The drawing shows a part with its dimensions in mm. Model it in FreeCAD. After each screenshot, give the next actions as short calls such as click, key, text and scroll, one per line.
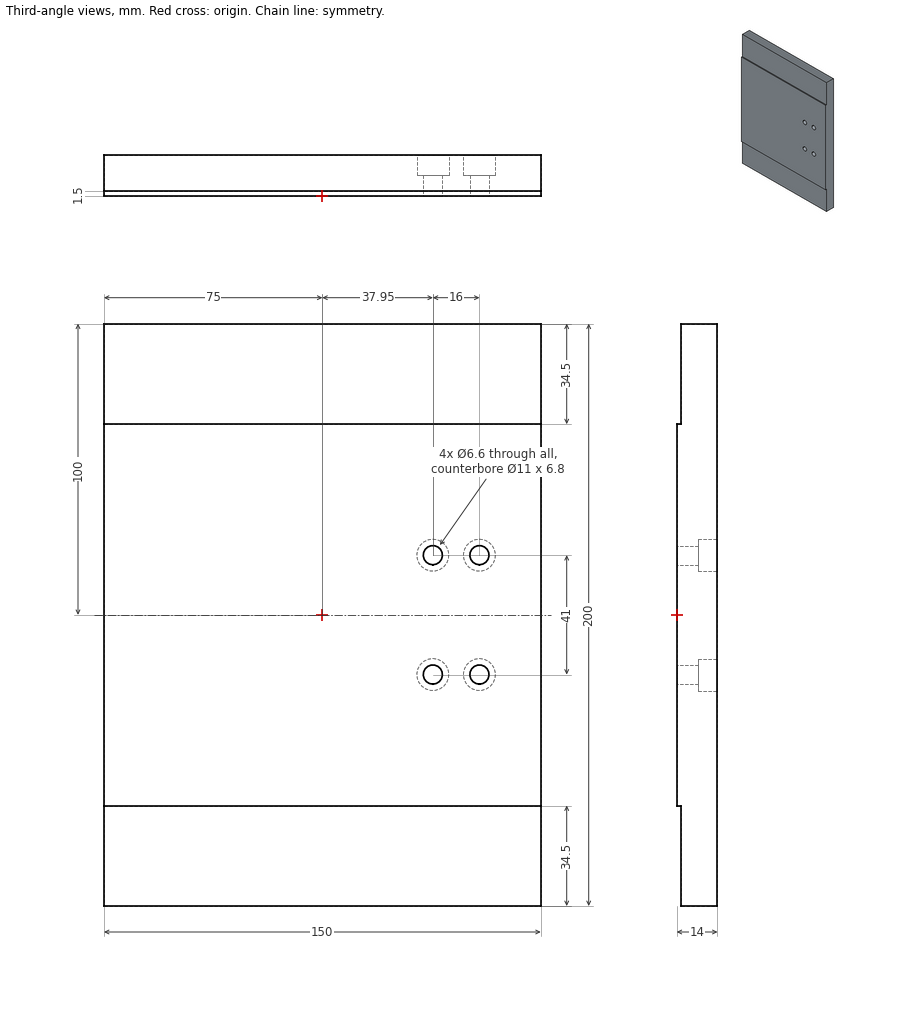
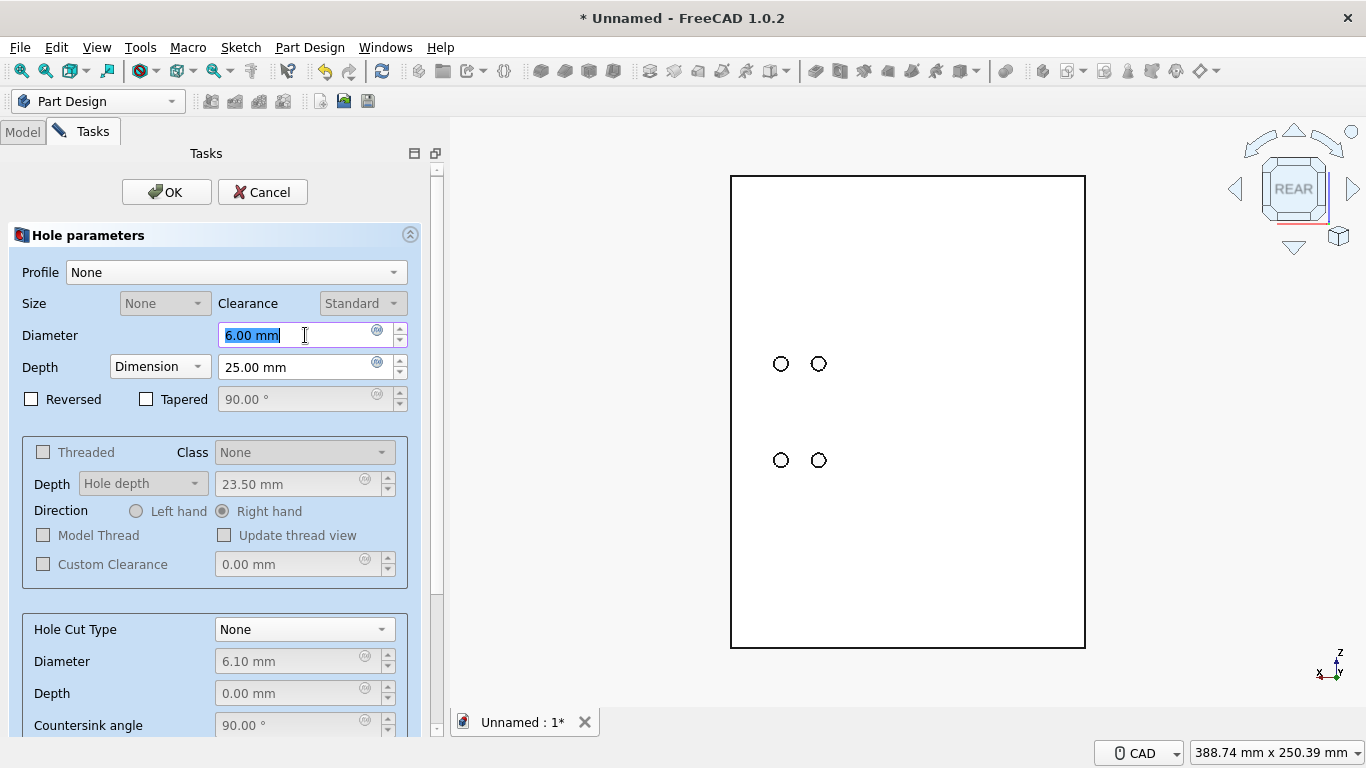
text(6.6)
key(Tab)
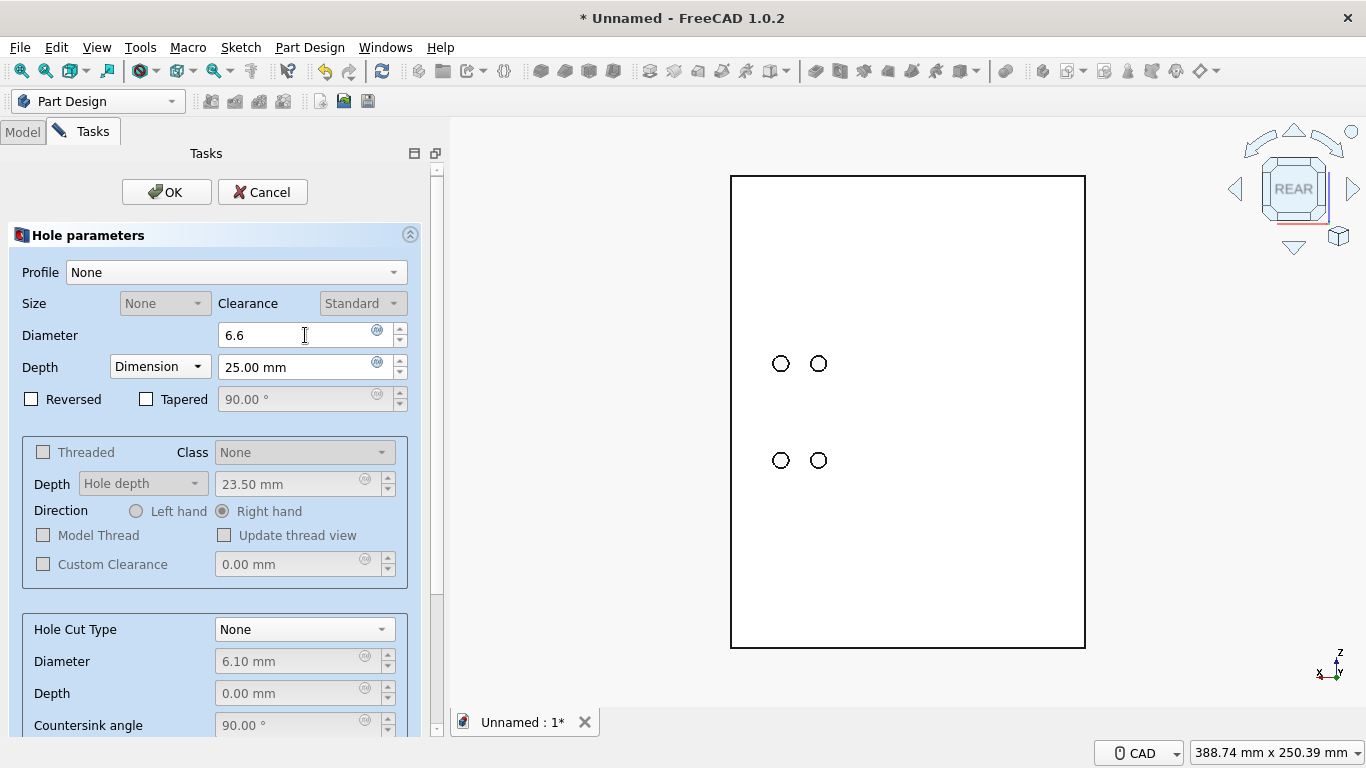
click(161, 366)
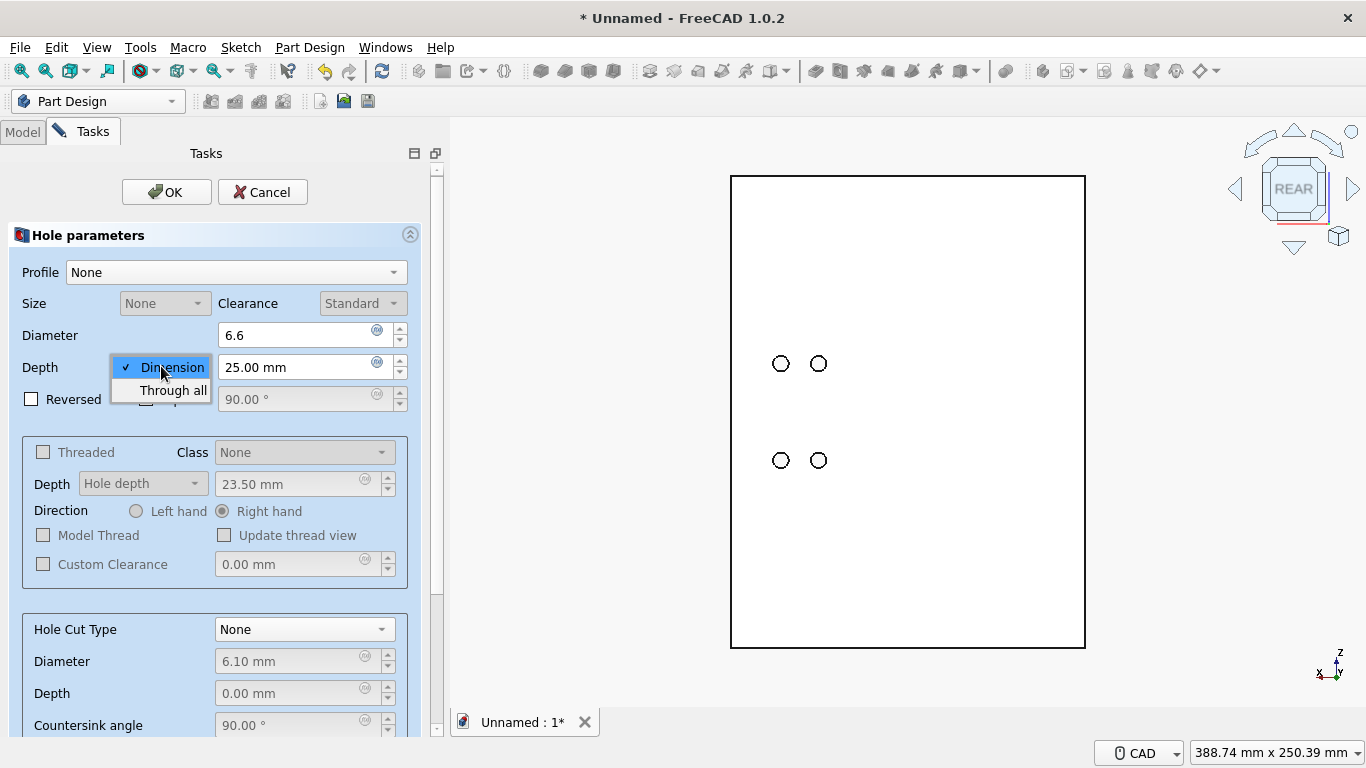
click(160, 390)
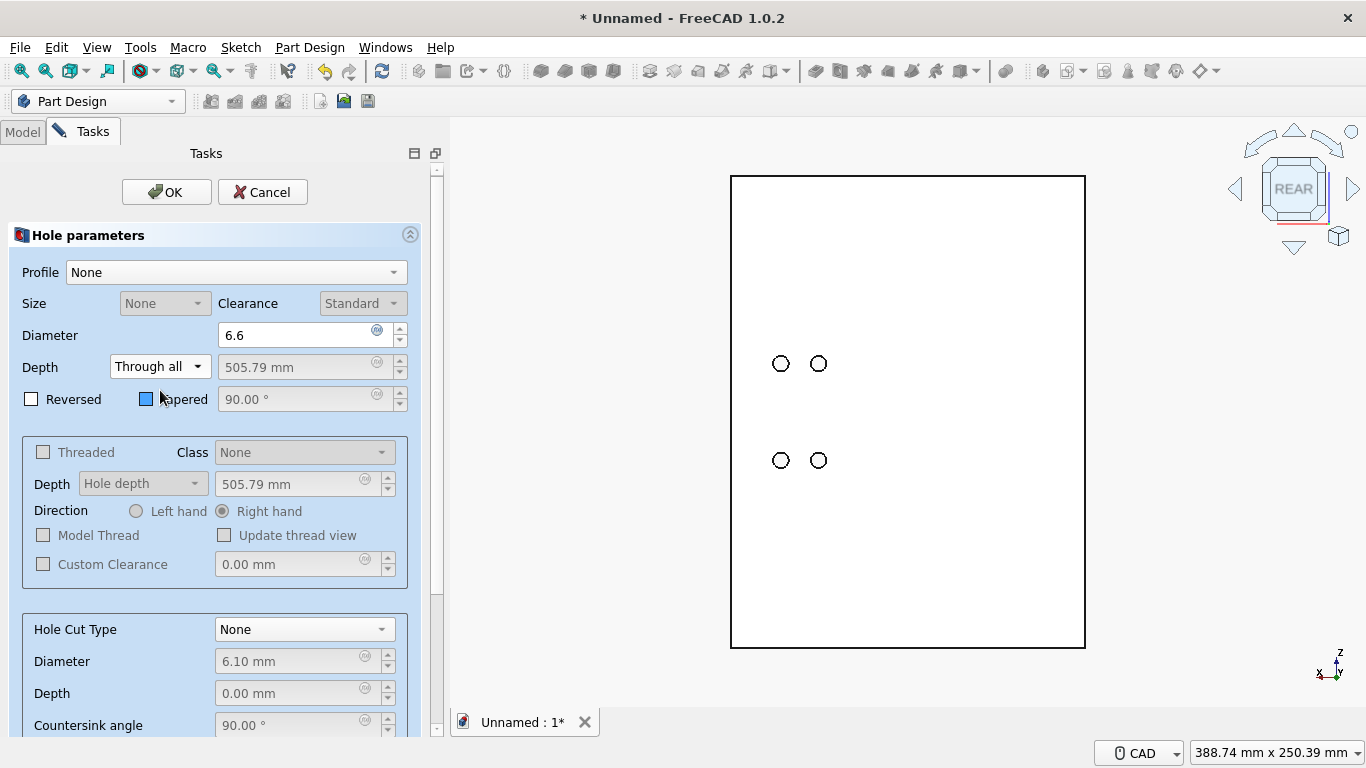
click(306, 630)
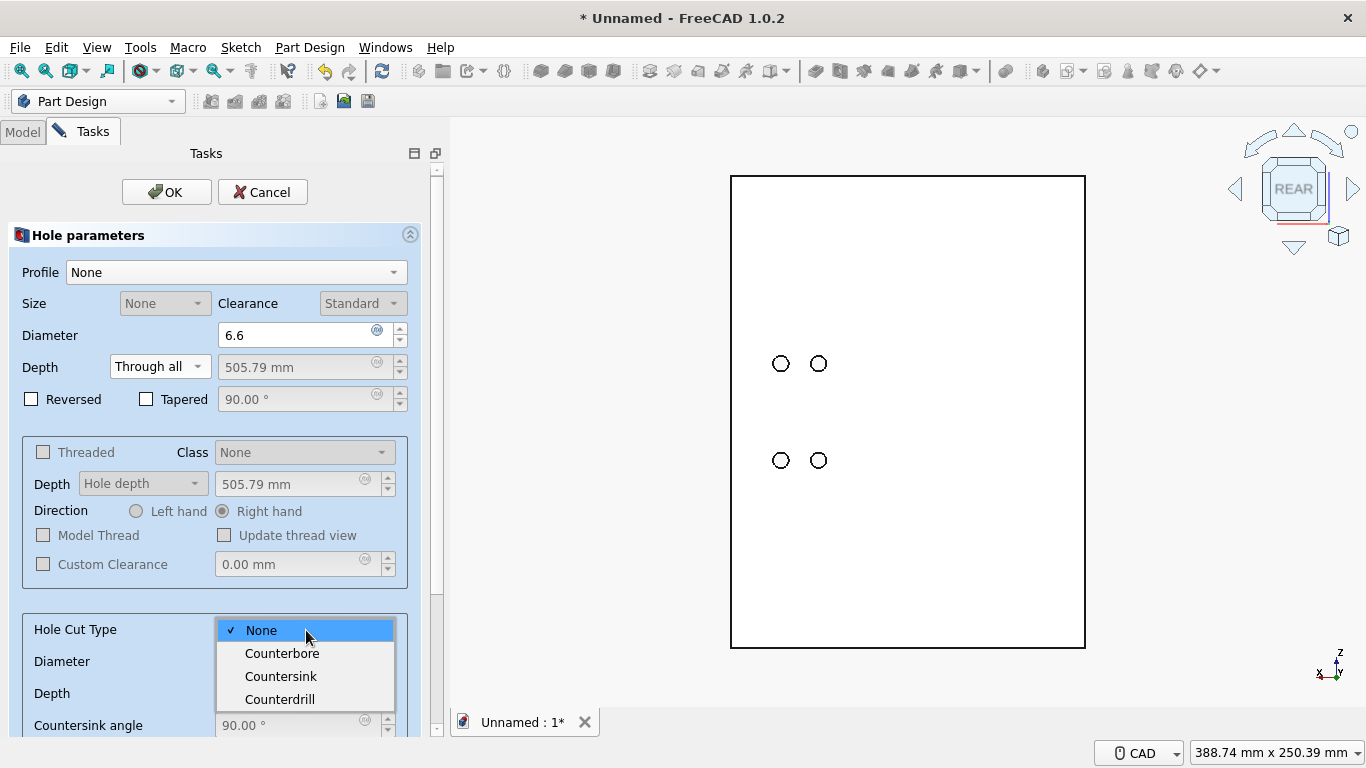
click(304, 654)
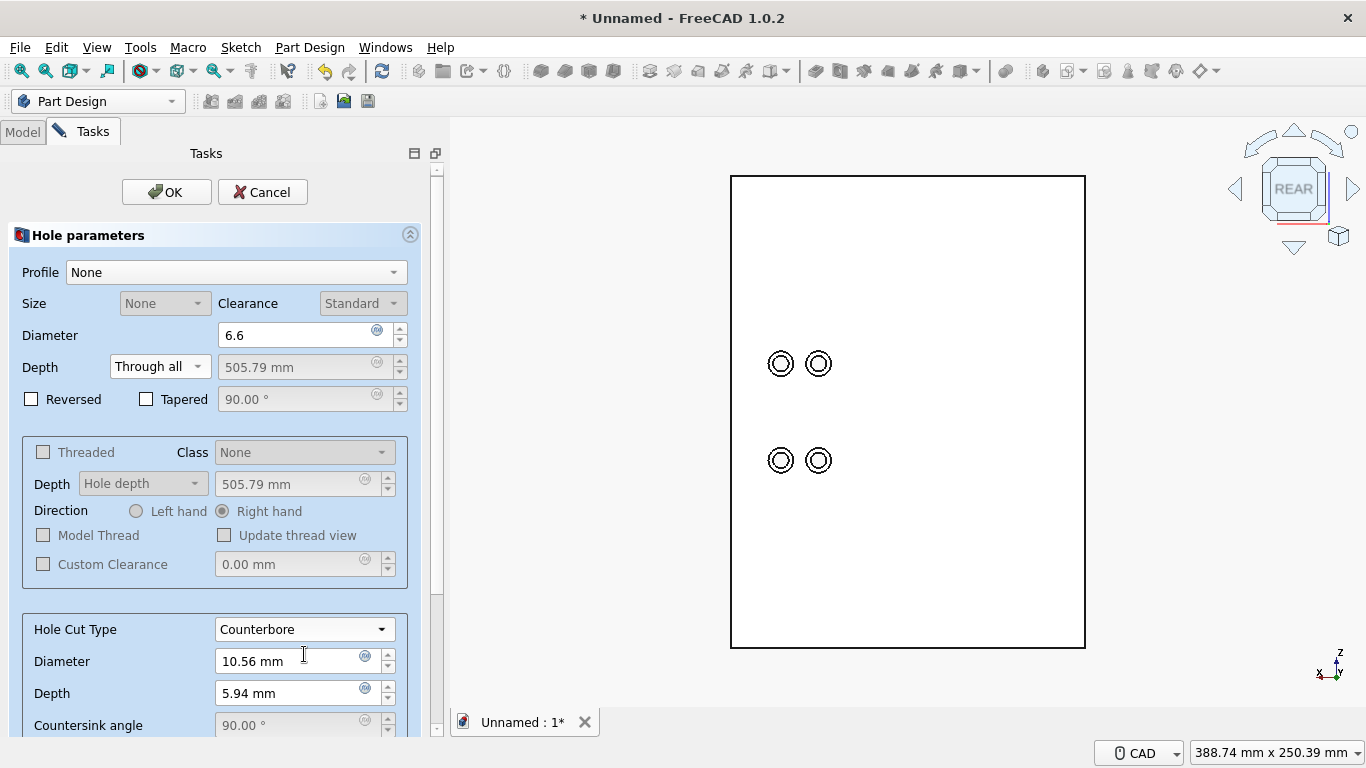
triple_click(298, 661)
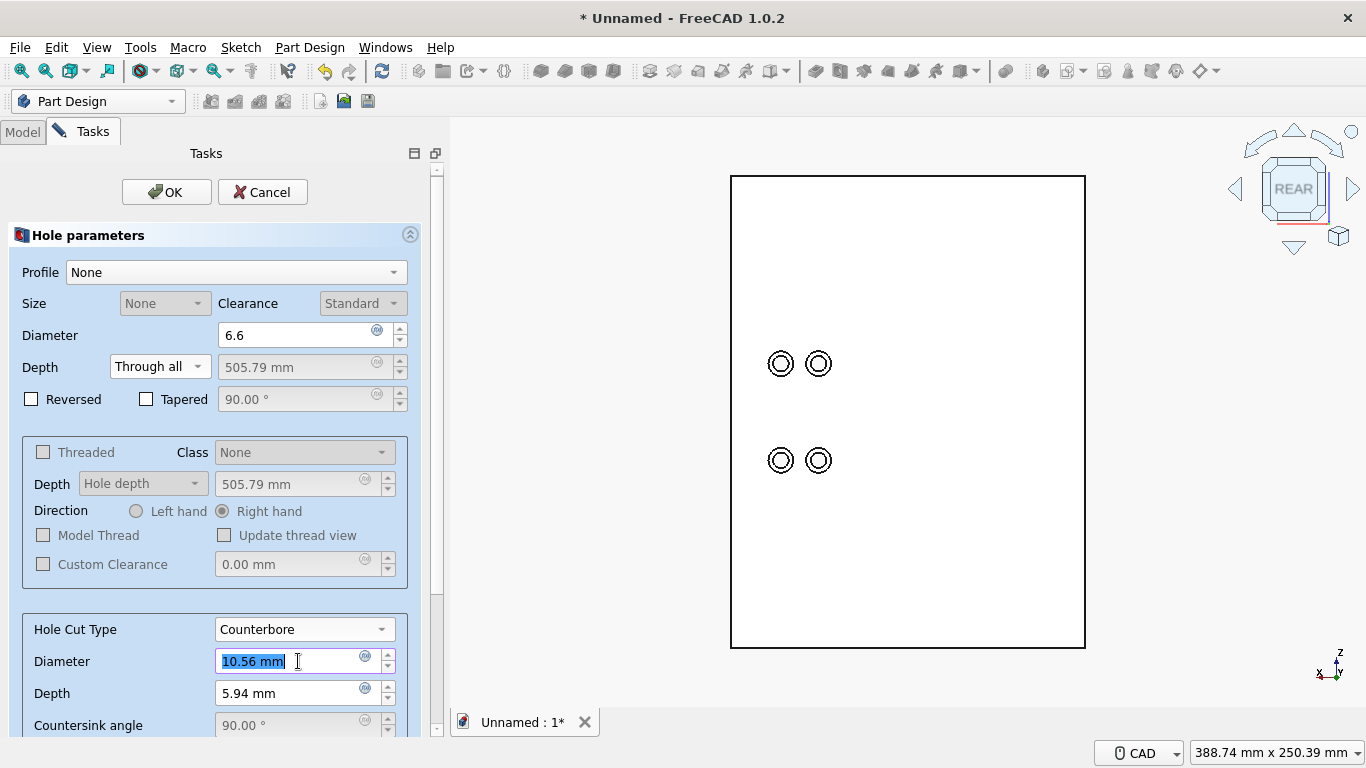
text(11)
key(Tab)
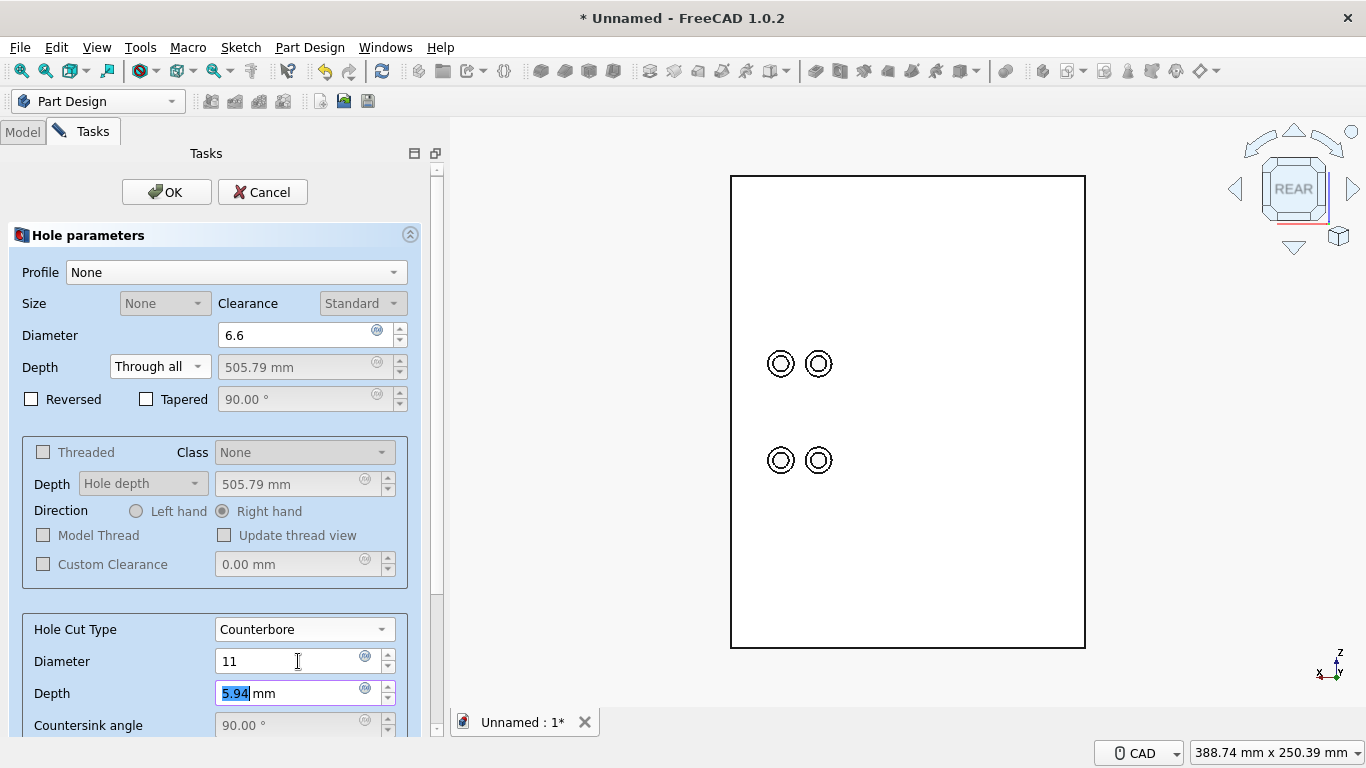
text(6.8)
key(Tab)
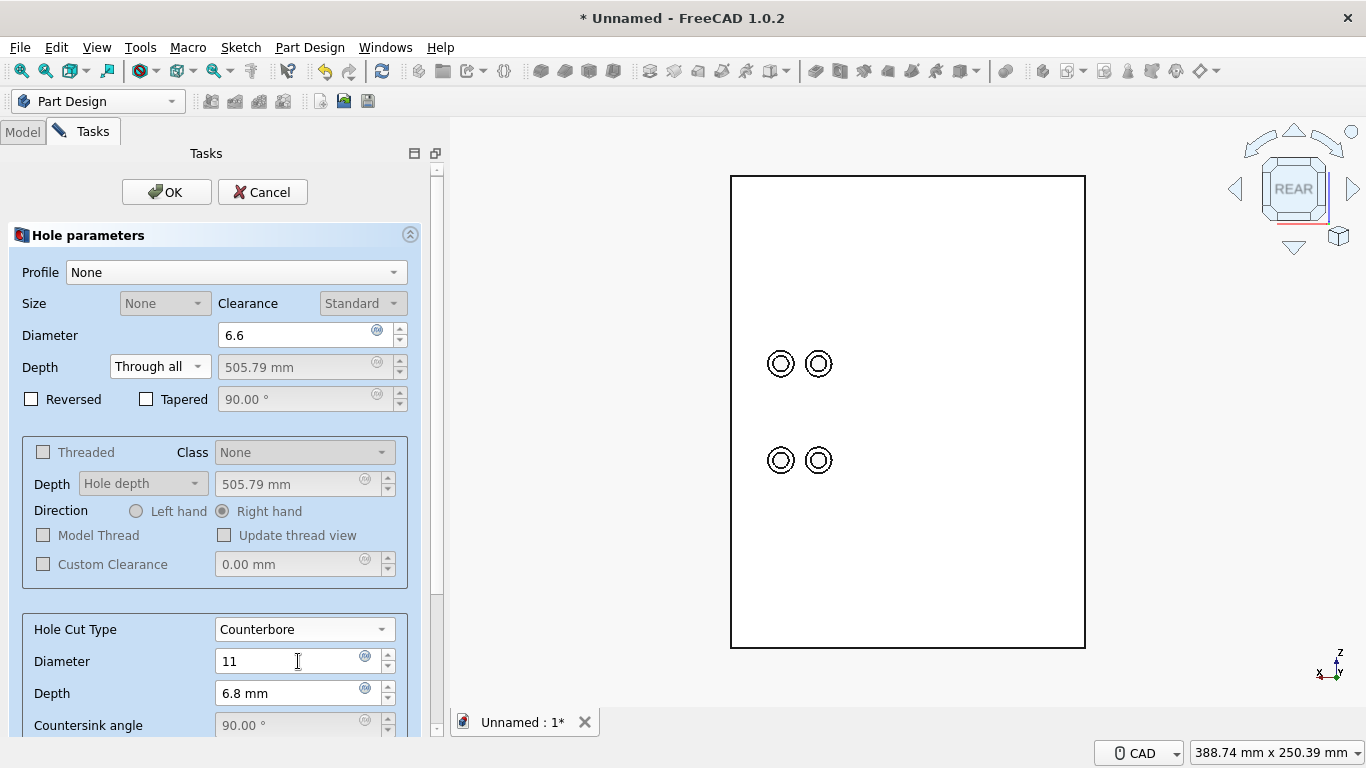
click(167, 192)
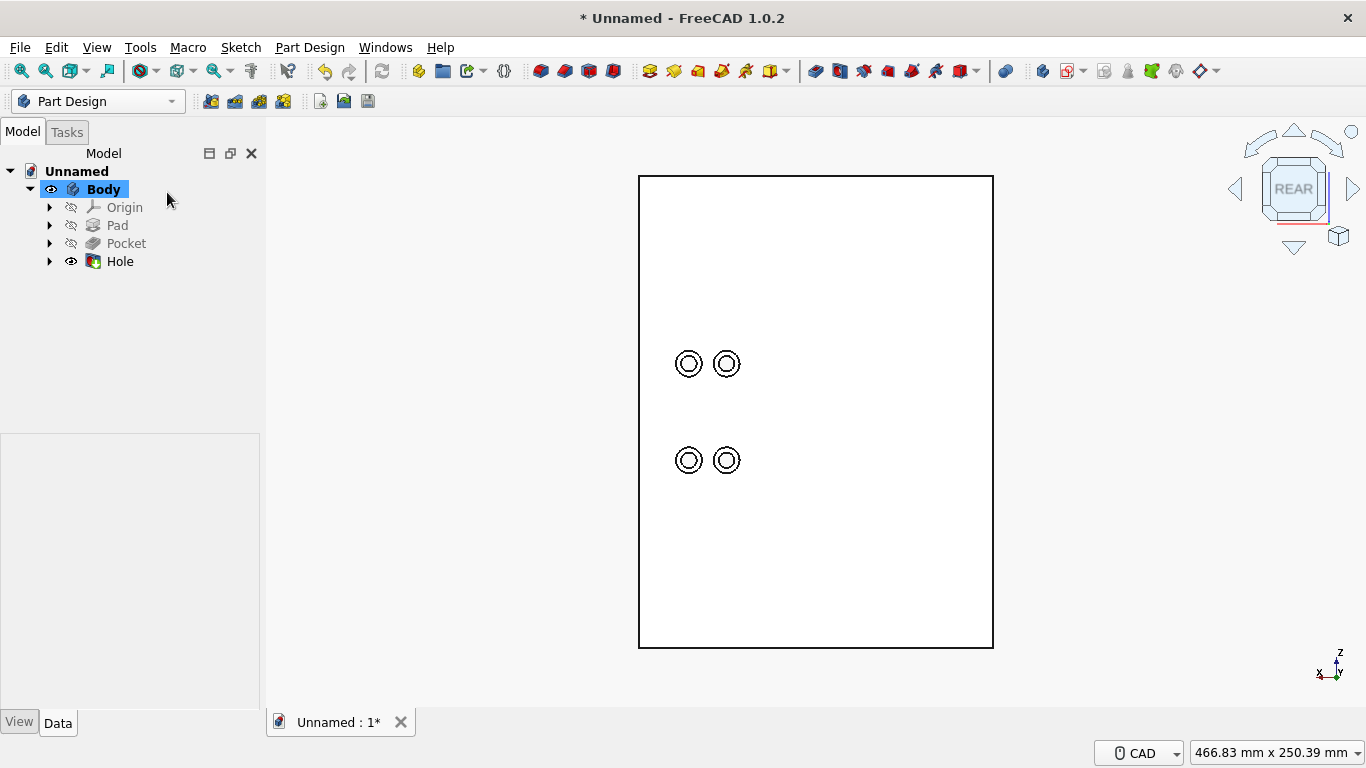
key(0)